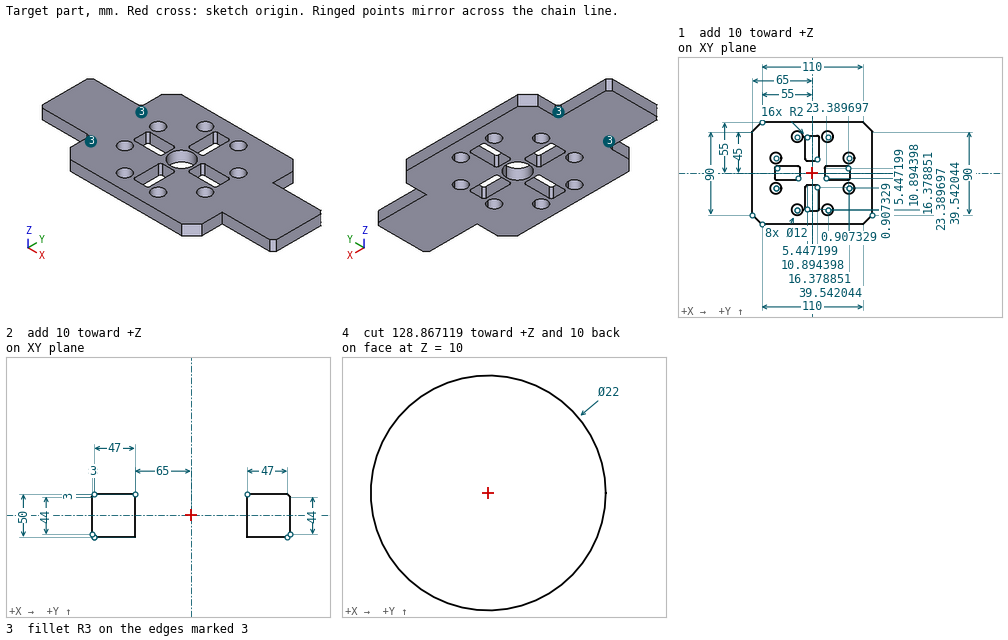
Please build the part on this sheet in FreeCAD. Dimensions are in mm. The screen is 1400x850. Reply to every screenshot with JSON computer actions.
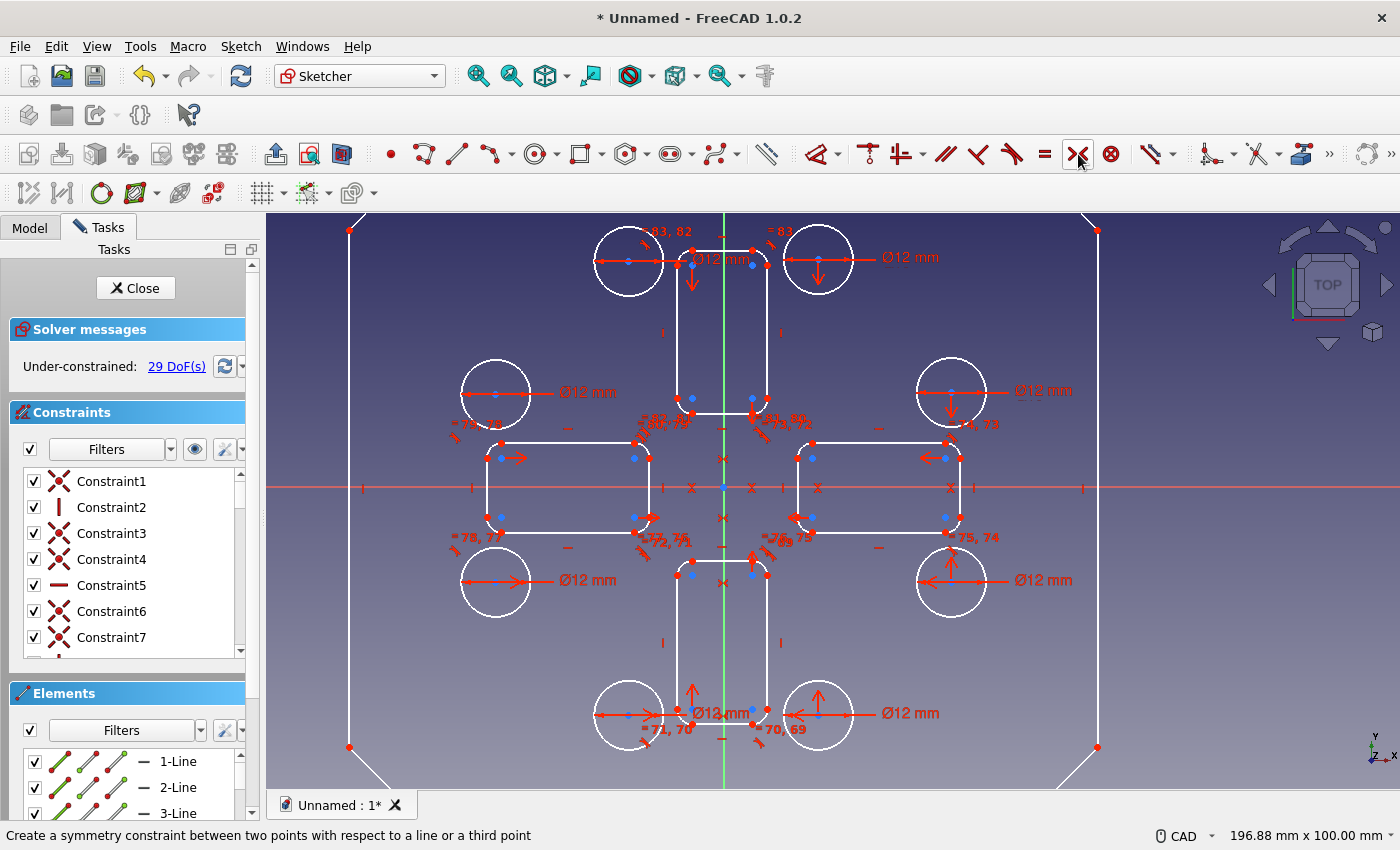
{"action": "left_click", "coordinate": [496, 582]}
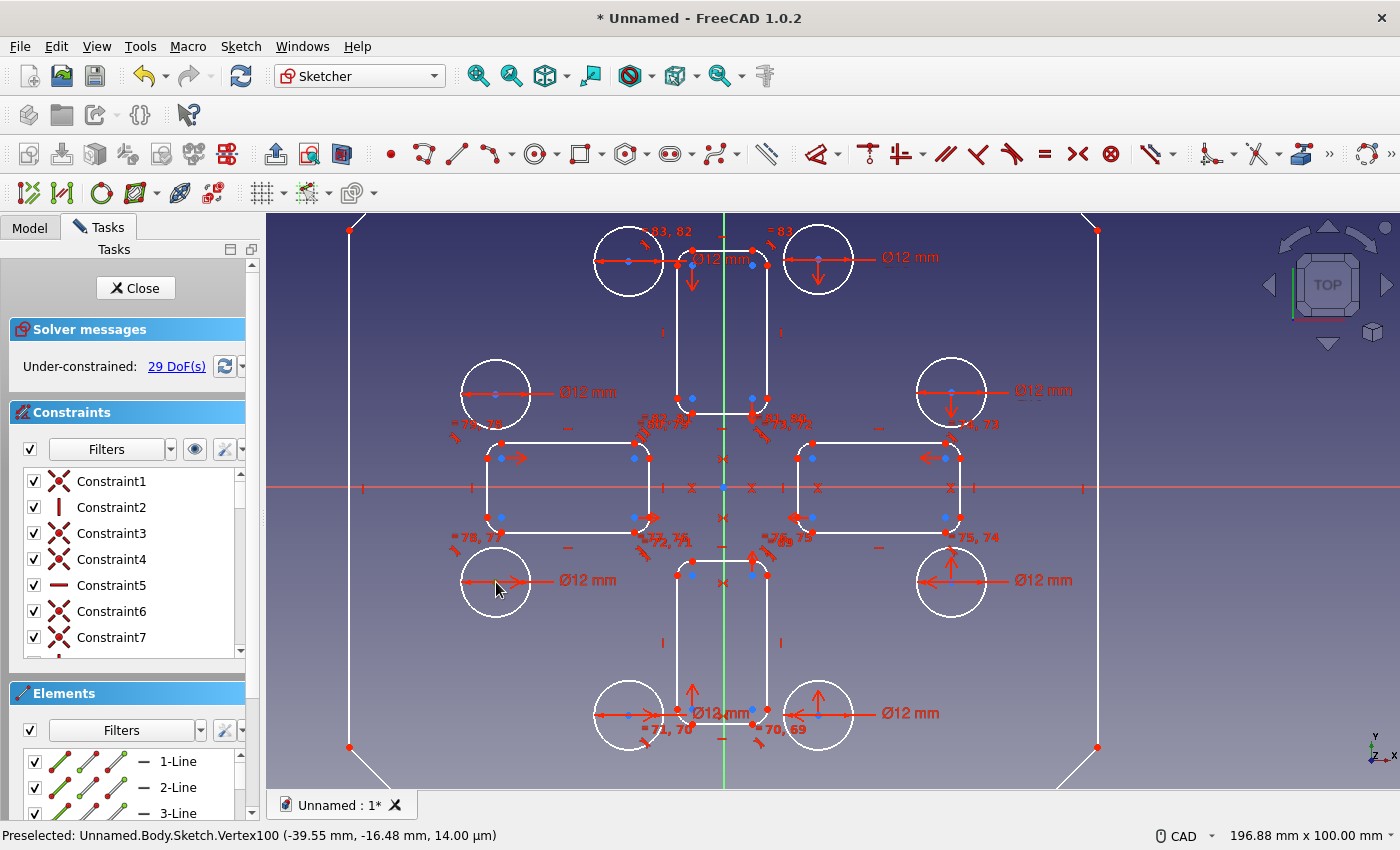
{"action": "left_click", "coordinate": [496, 394]}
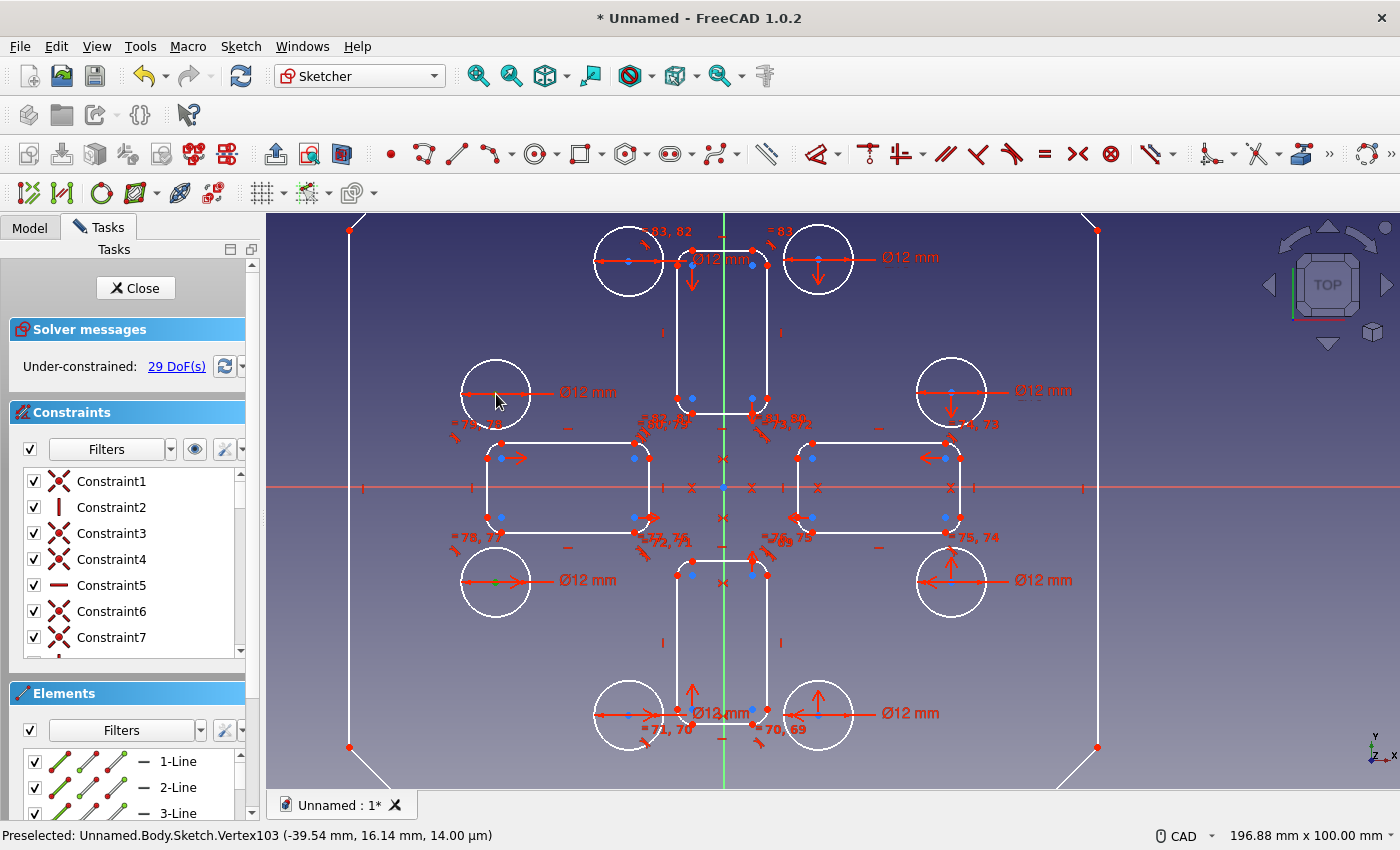
{"action": "left_click", "coordinate": [428, 487]}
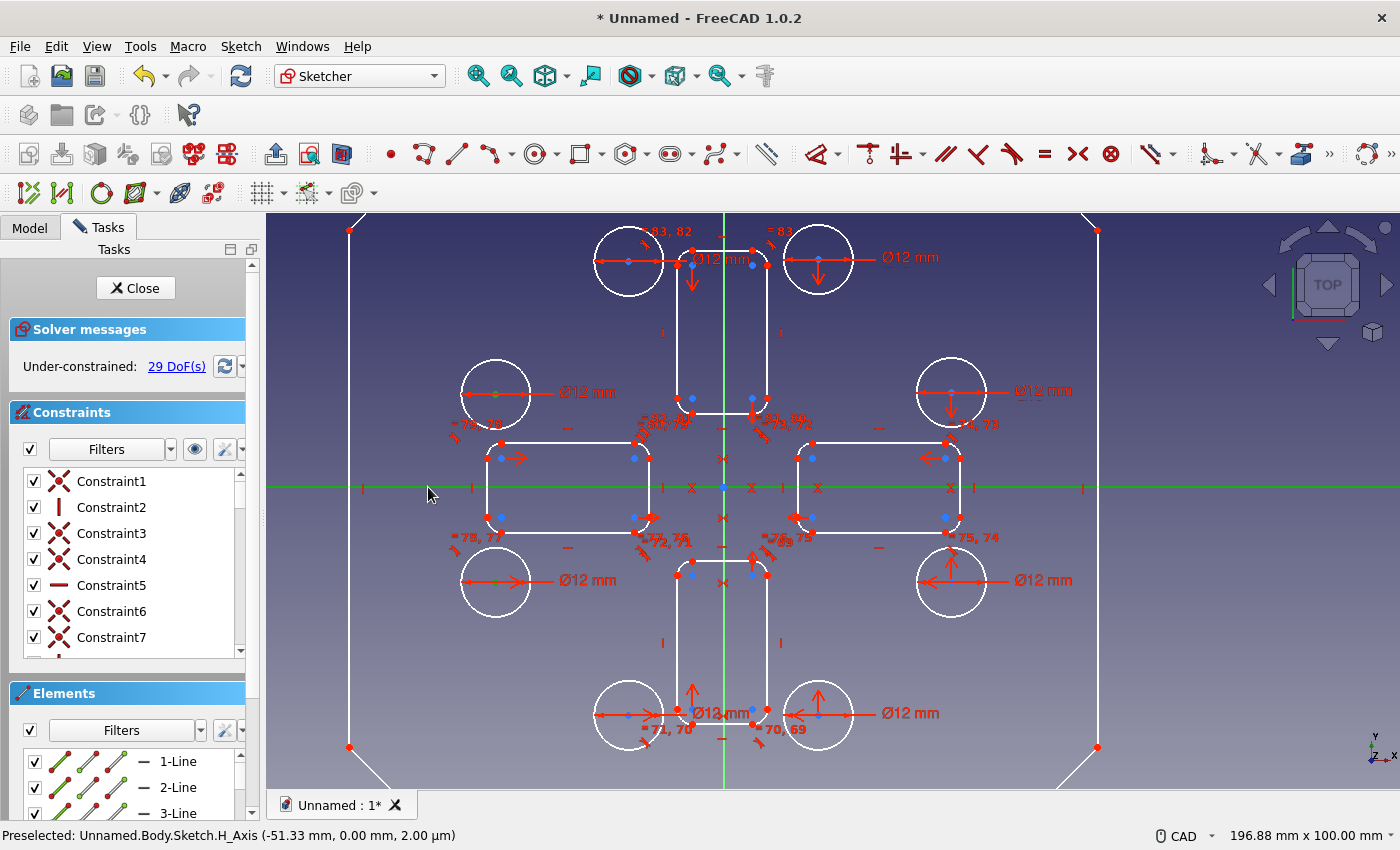
{"action": "left_click", "coordinate": [1078, 154]}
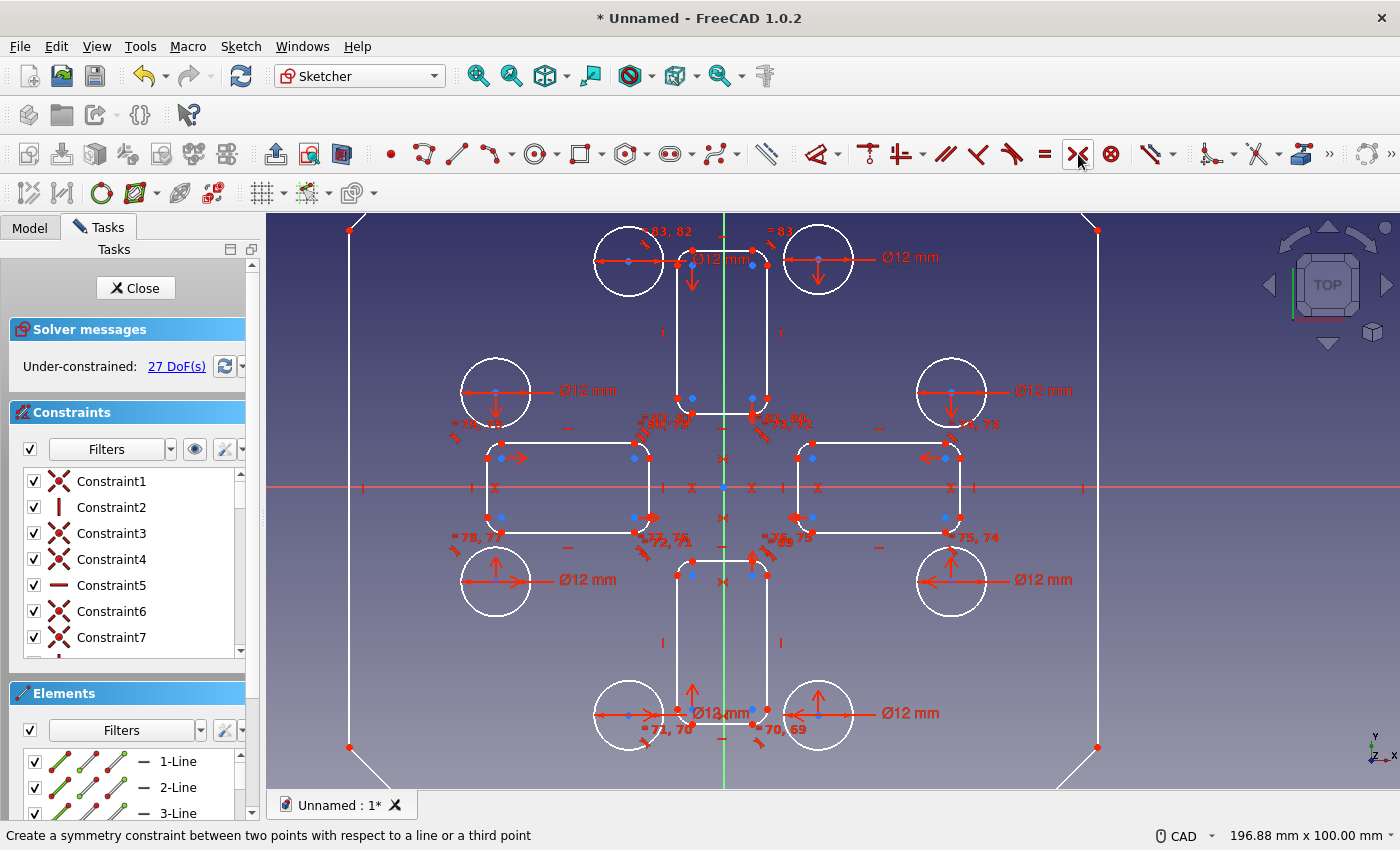
{"action": "left_click", "coordinate": [629, 715]}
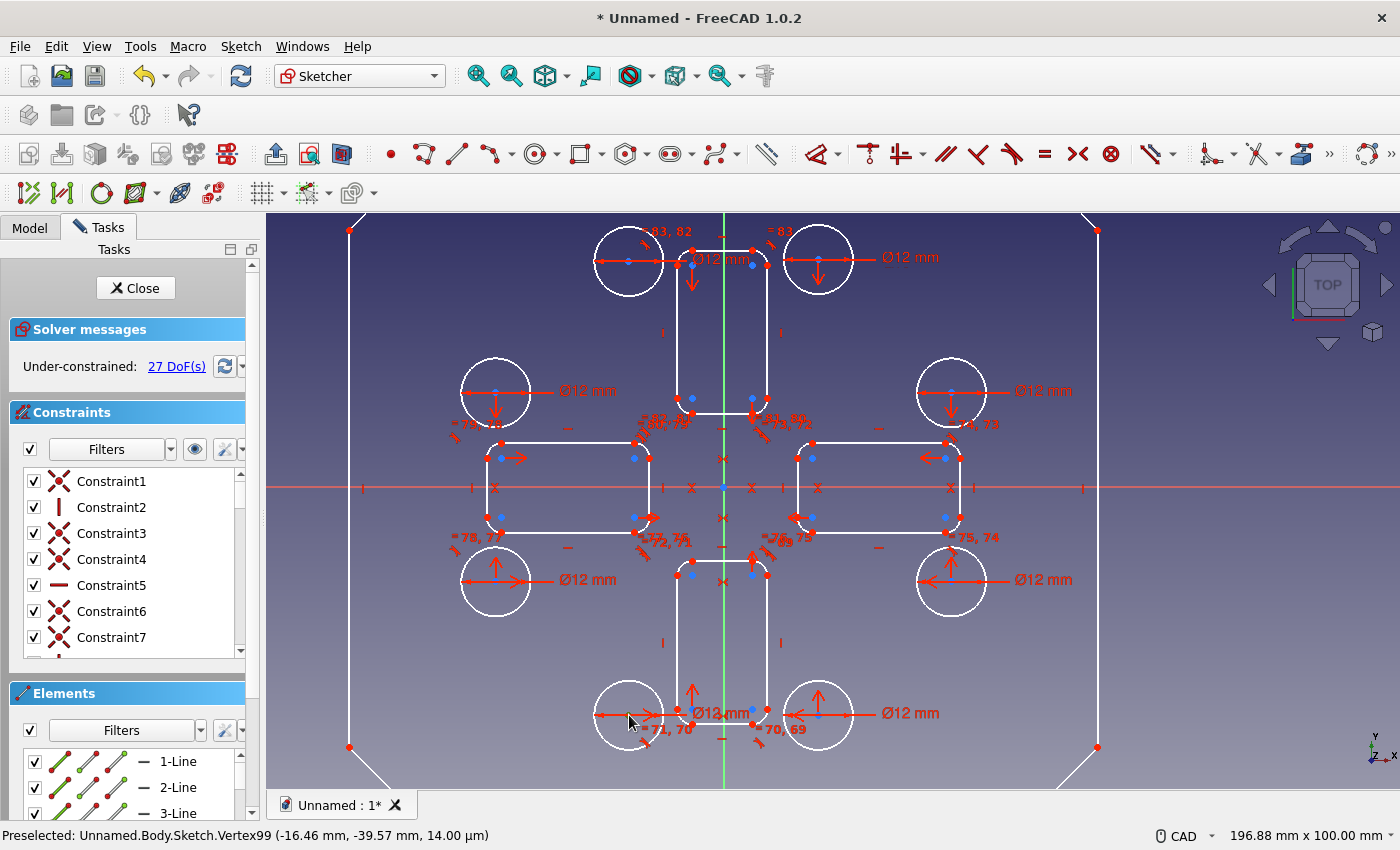
{"action": "left_click", "coordinate": [629, 261]}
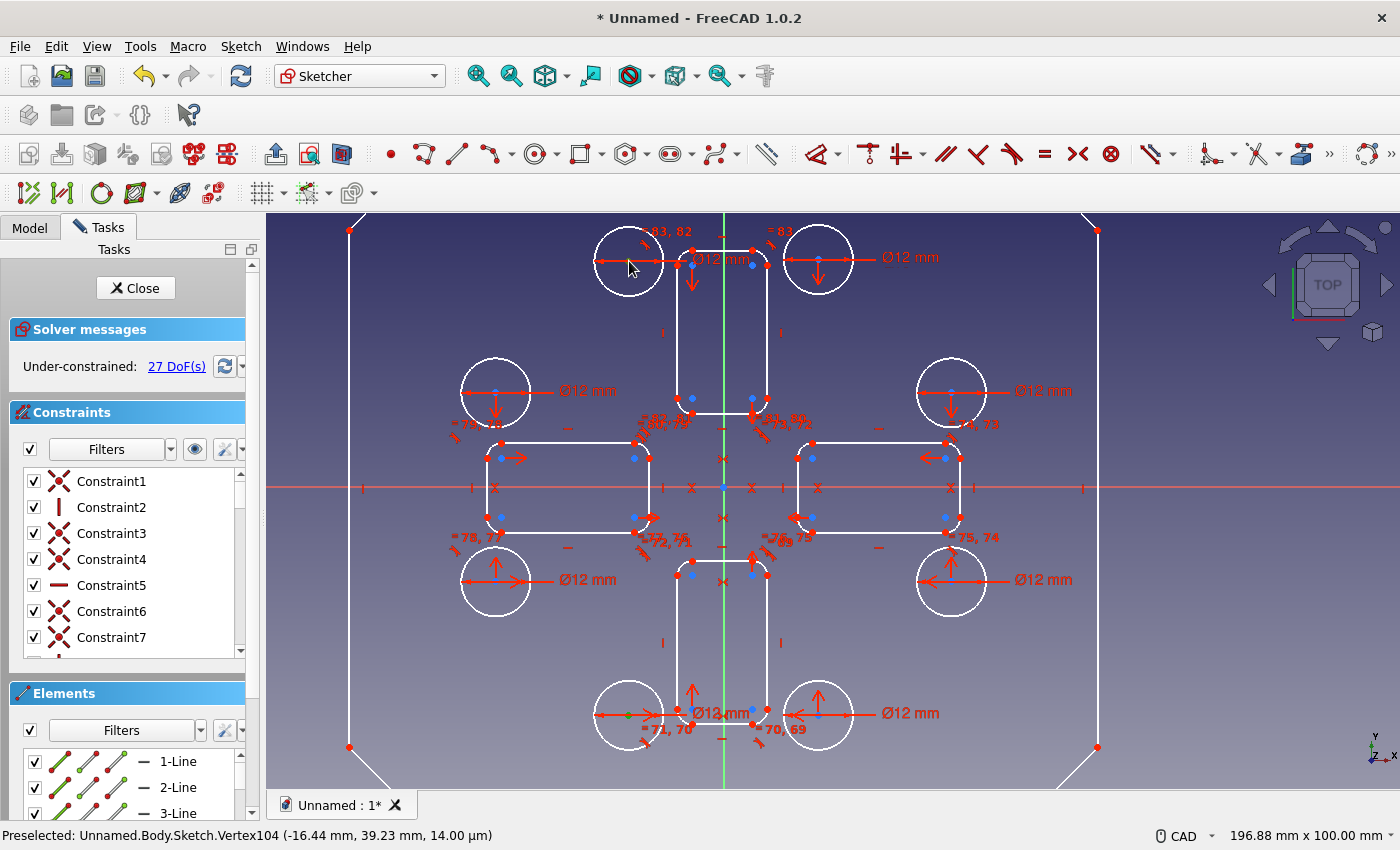
{"action": "left_click", "coordinate": [428, 487]}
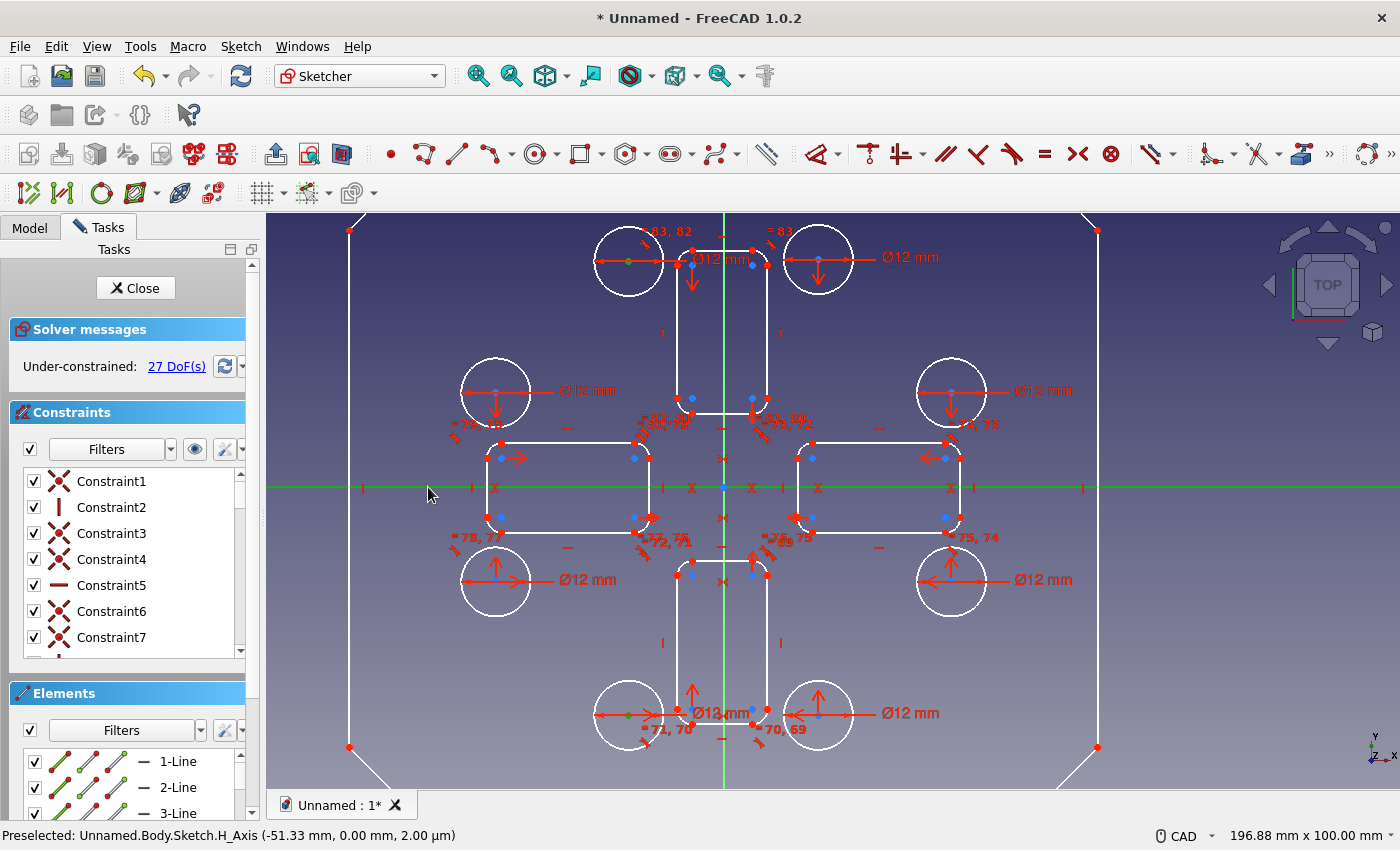
{"action": "left_click", "coordinate": [1078, 154]}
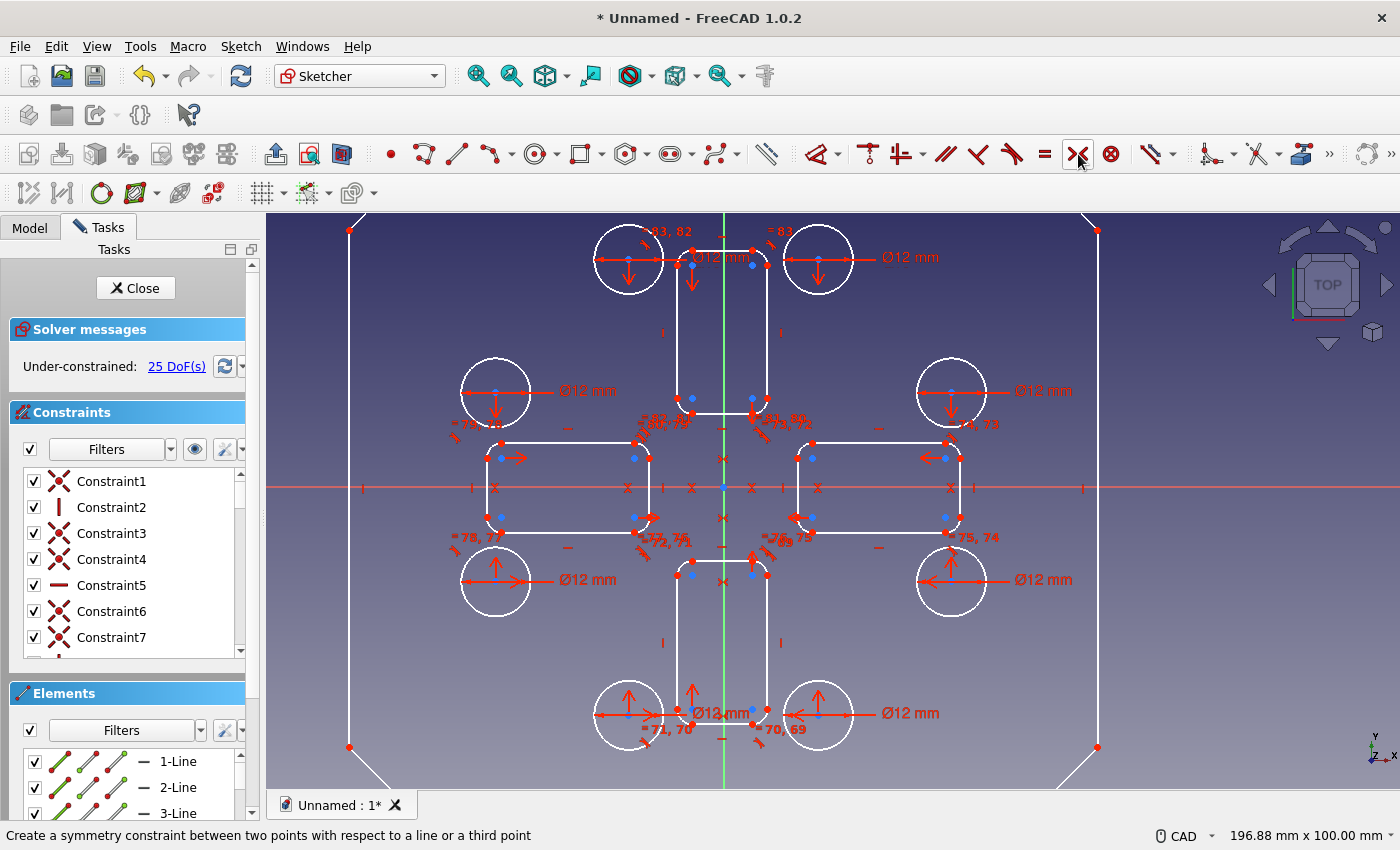
{"action": "scroll", "coordinate": [814, 517], "scroll_direction": "down", "scroll_amount": 3}